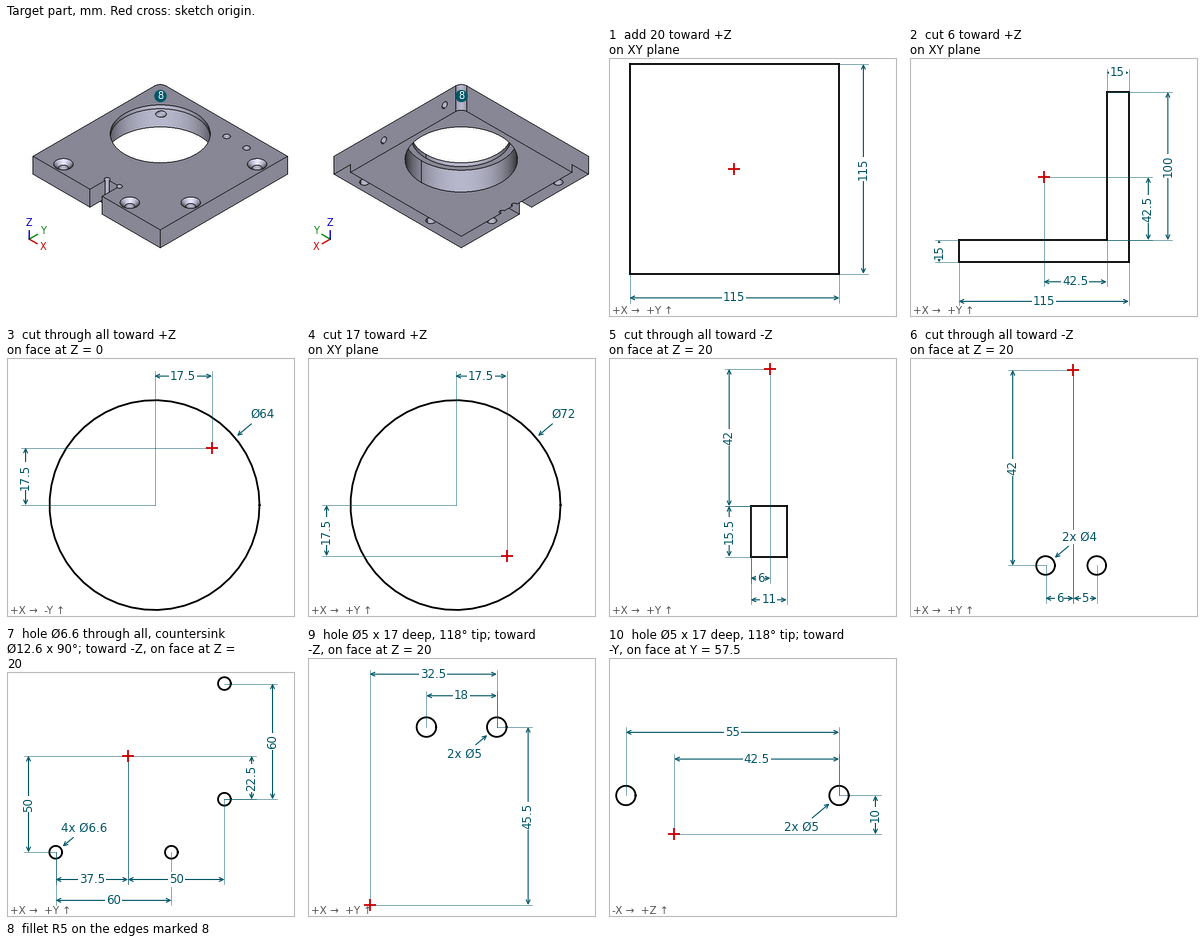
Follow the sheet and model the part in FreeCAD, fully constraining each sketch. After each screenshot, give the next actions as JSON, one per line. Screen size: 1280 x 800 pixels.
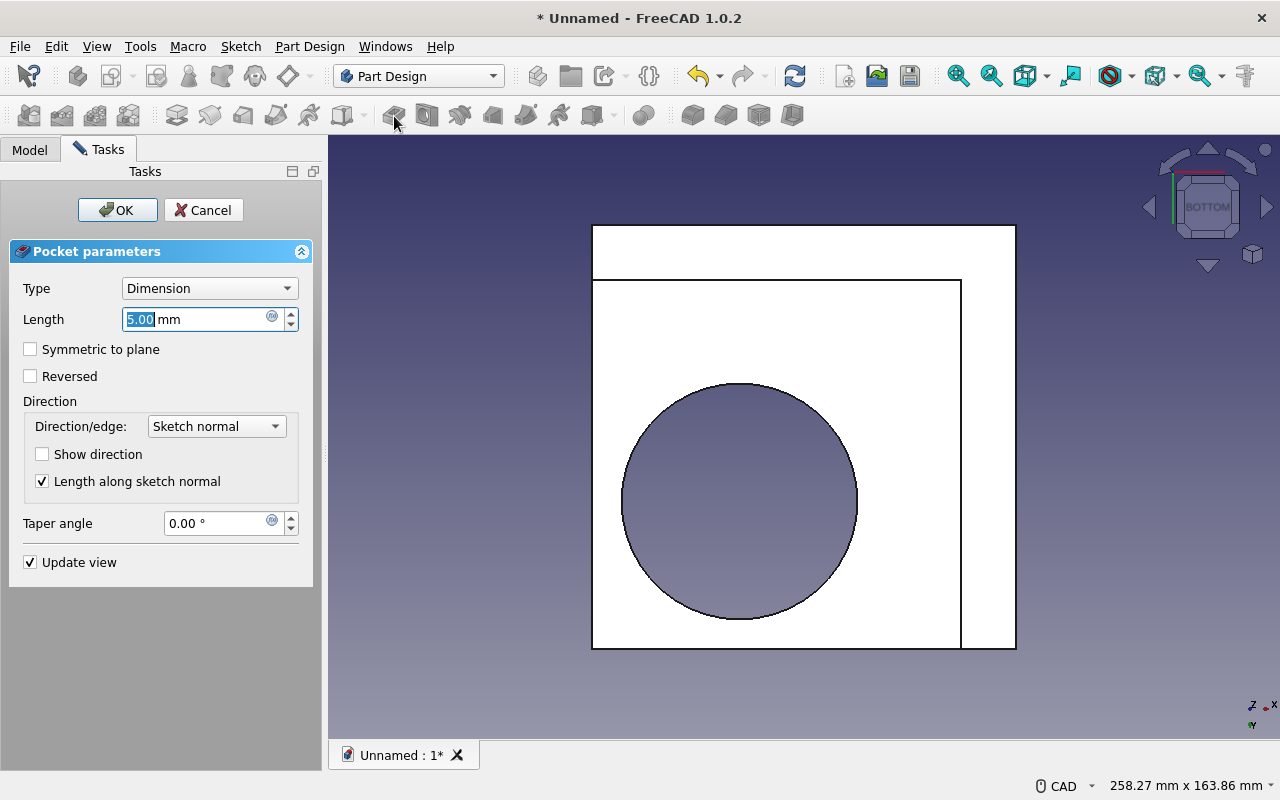
{"action": "type", "text": "17"}
{"action": "key", "text": "Tab"}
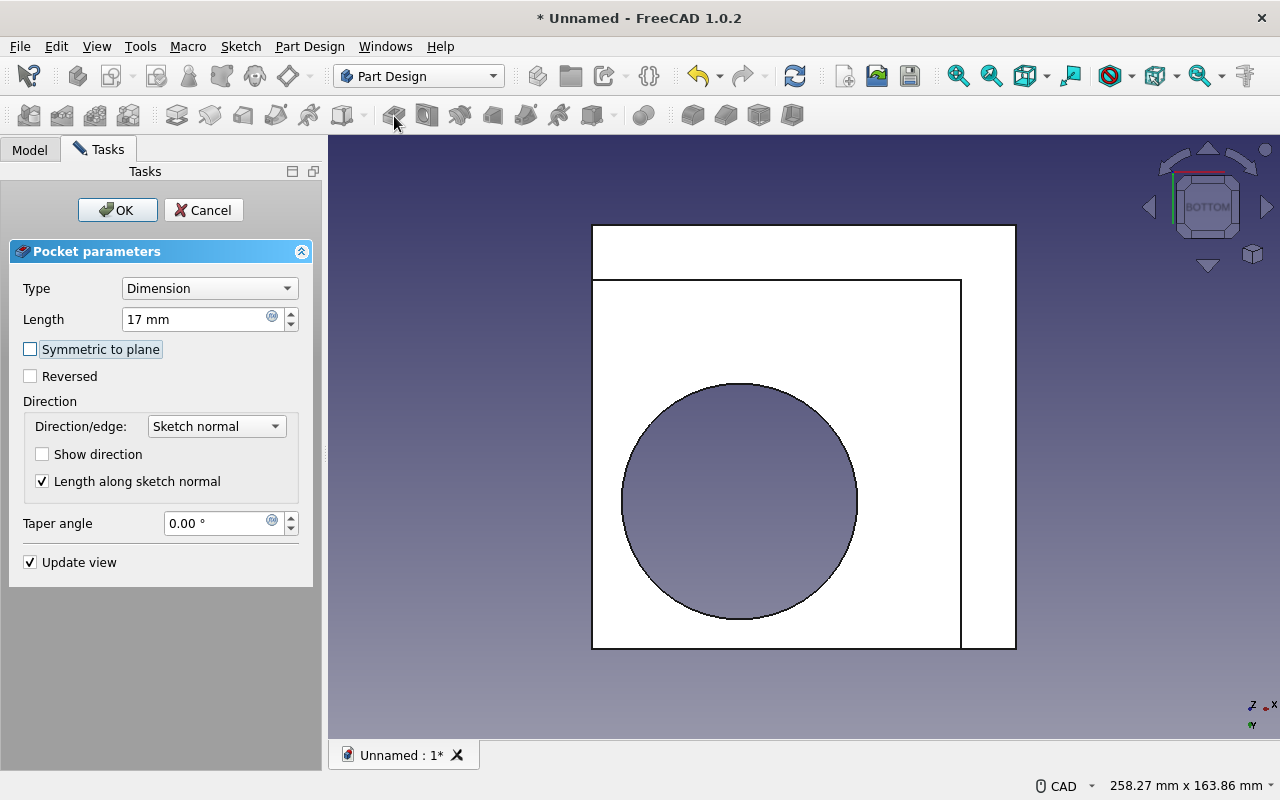
{"action": "left_click", "coordinate": [31, 376]}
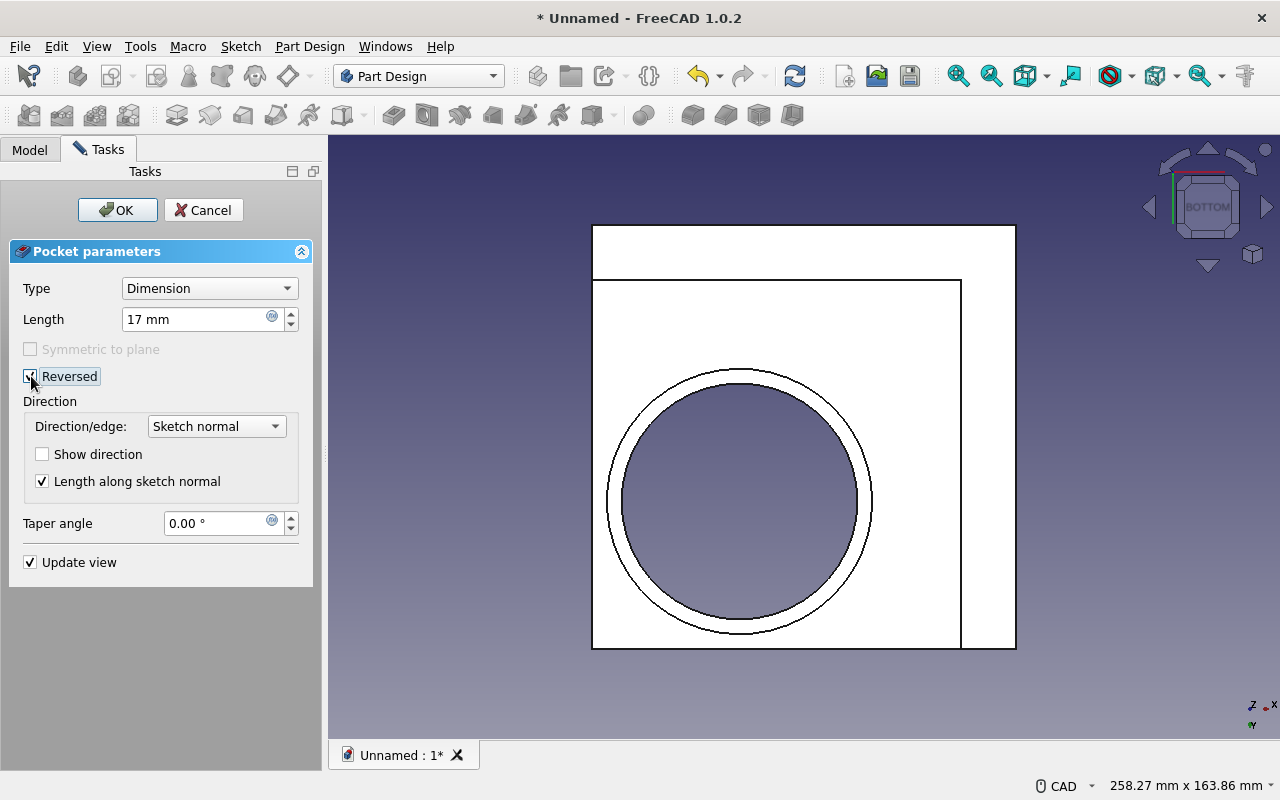
{"action": "left_click", "coordinate": [118, 210]}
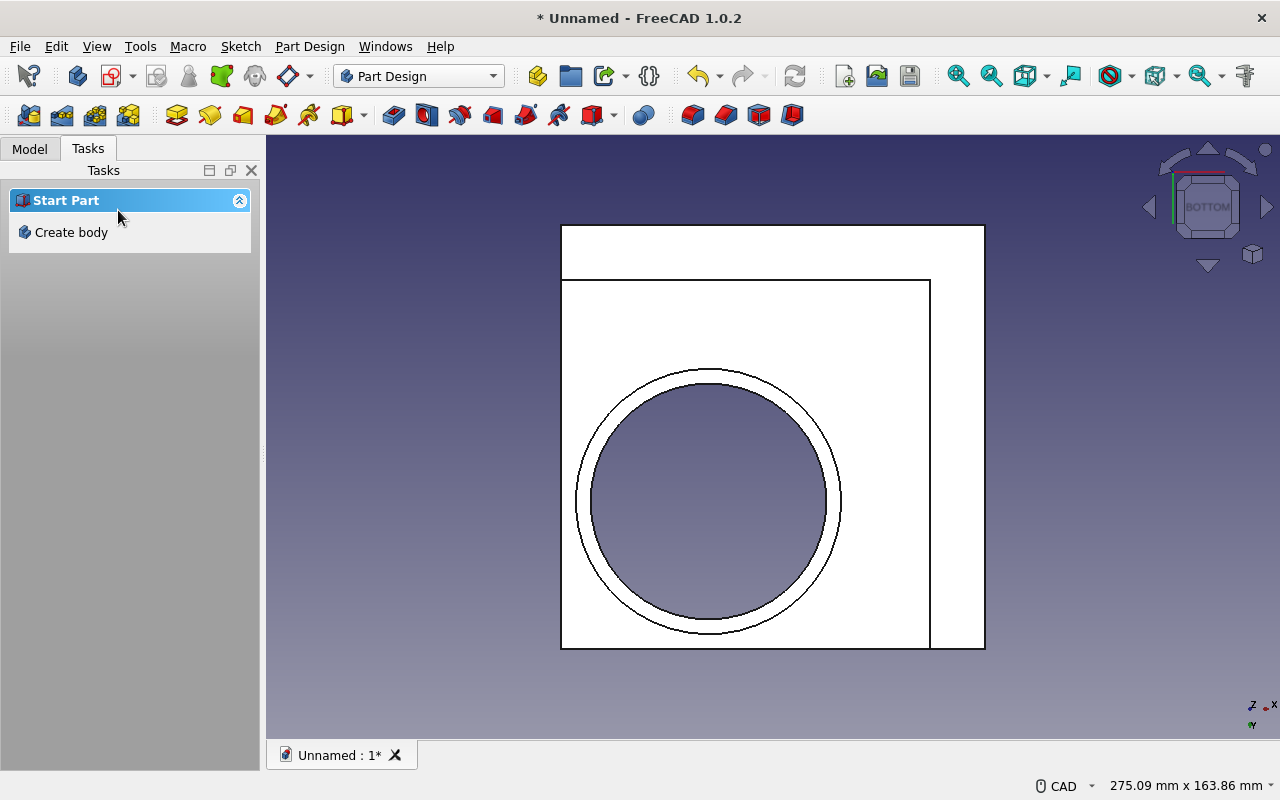
{"action": "key", "text": "0"}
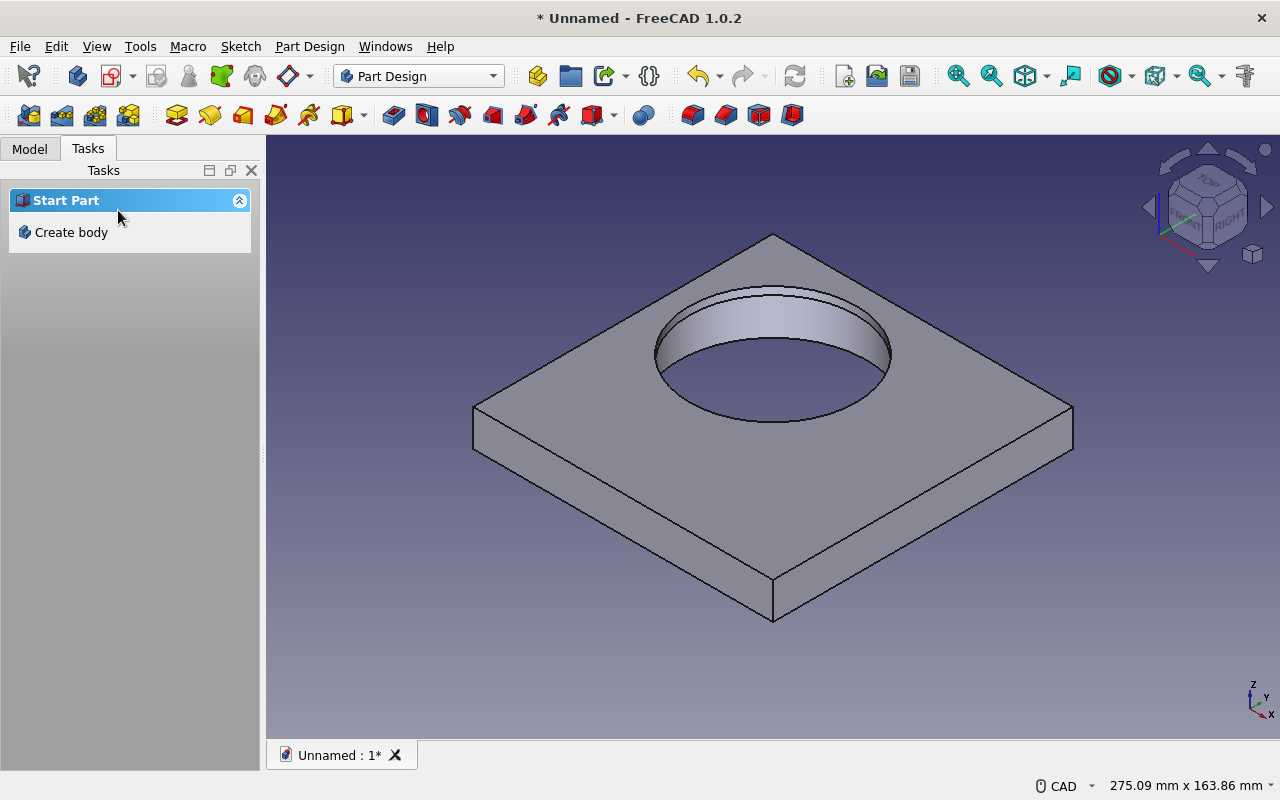
{"action": "left_click", "coordinate": [816, 480]}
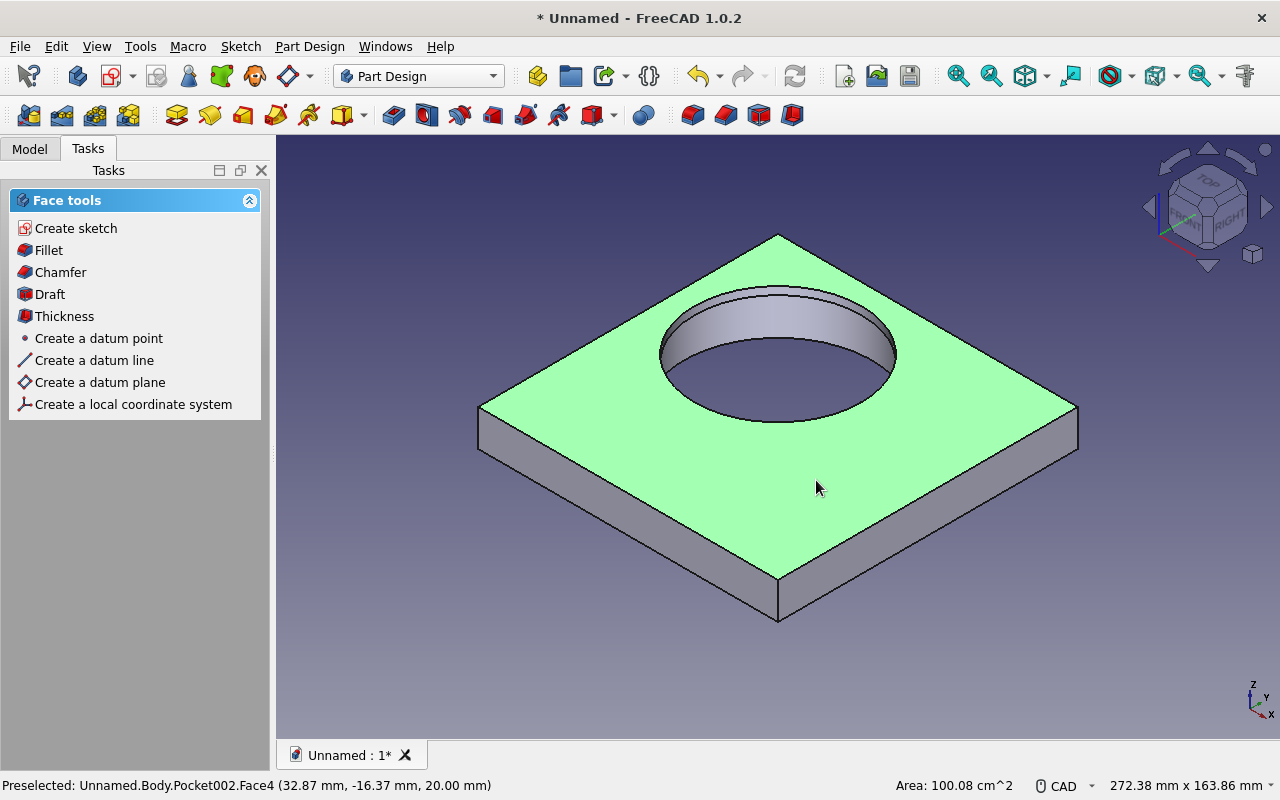
{"action": "left_click", "coordinate": [110, 76]}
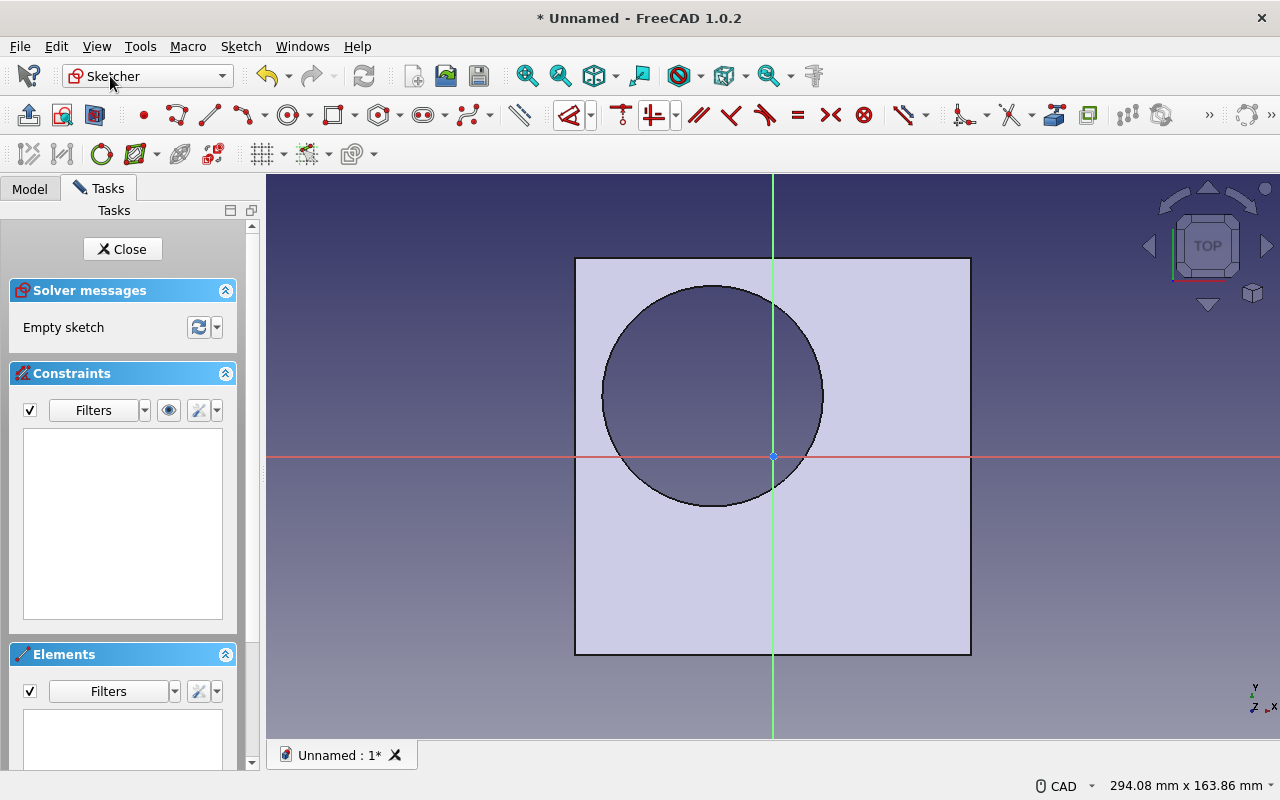
{"action": "scroll", "coordinate": [782, 655], "scroll_direction": "up", "scroll_amount": 10}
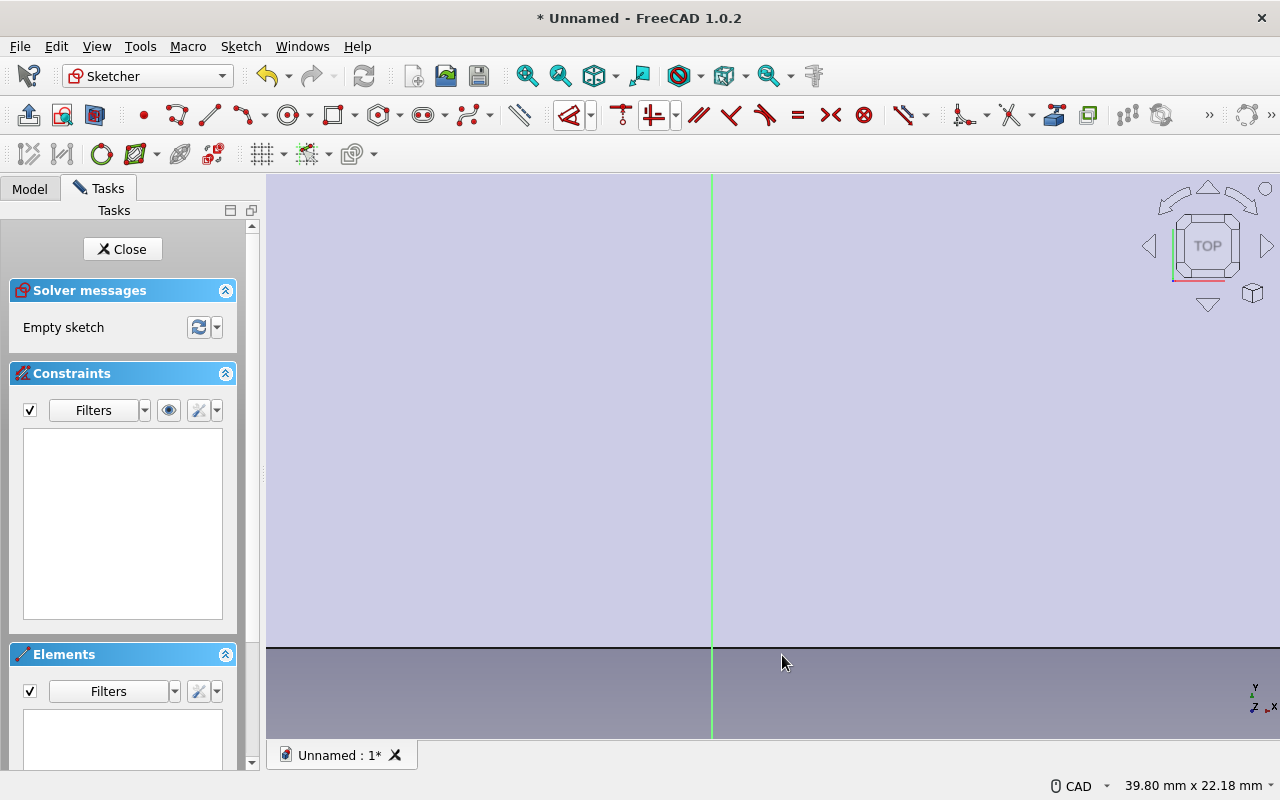
{"action": "key", "text": "g r"}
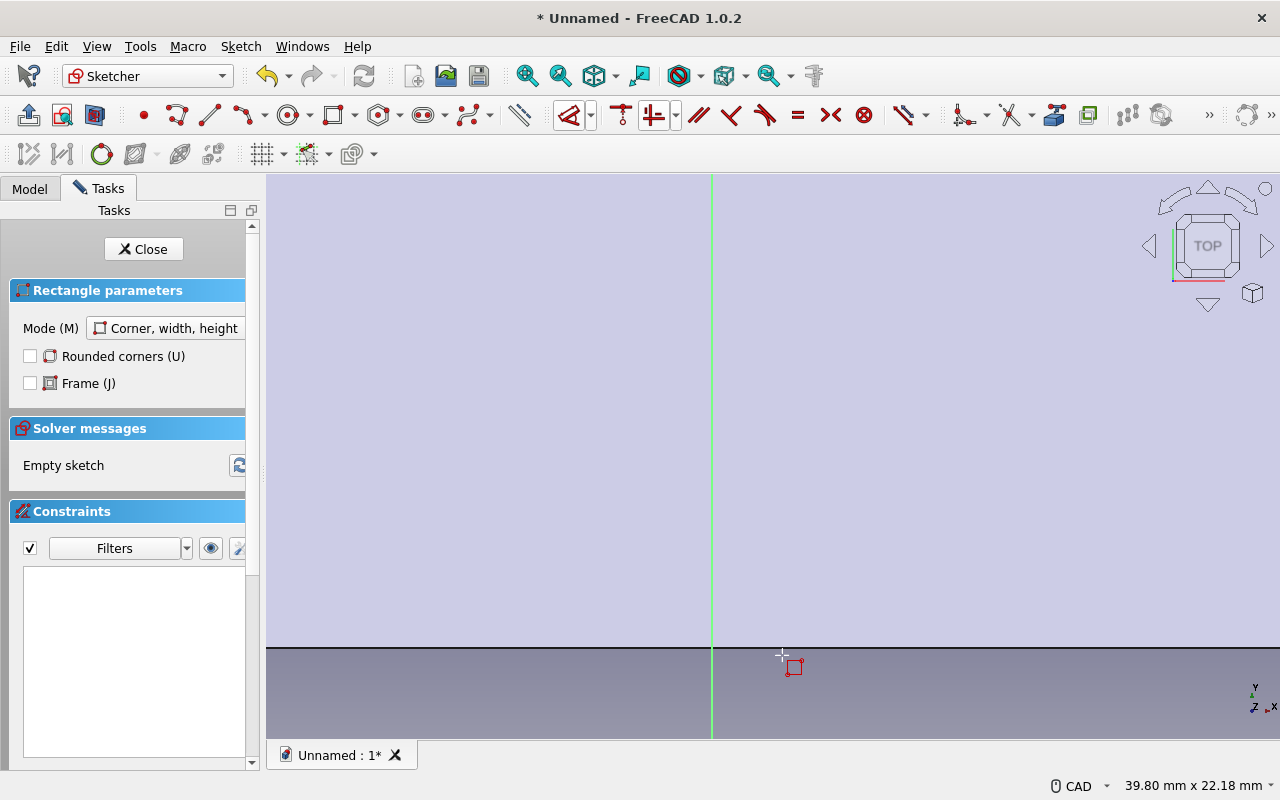
{"action": "left_click", "coordinate": [559, 253]}
{"action": "left_click", "coordinate": [840, 648]}
{"action": "key", "text": "Escape"}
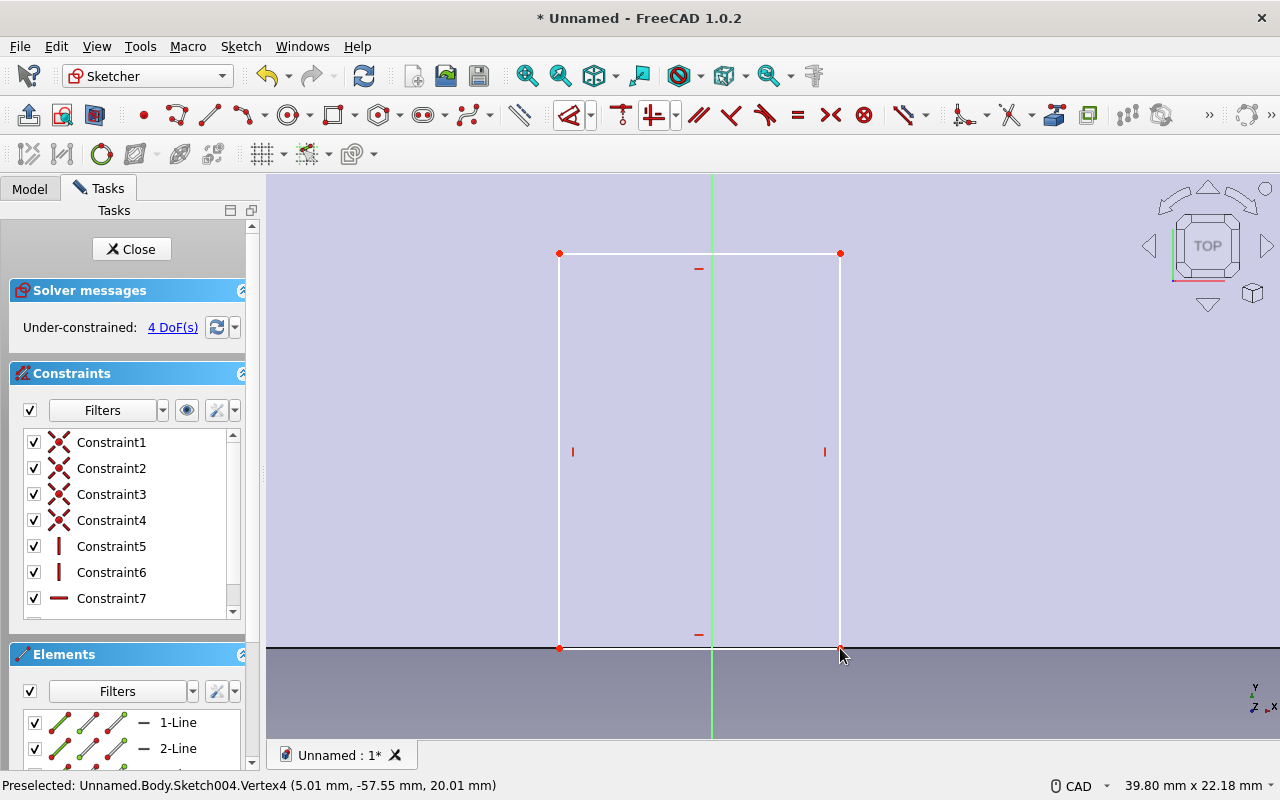
{"action": "left_click", "coordinate": [643, 649]}